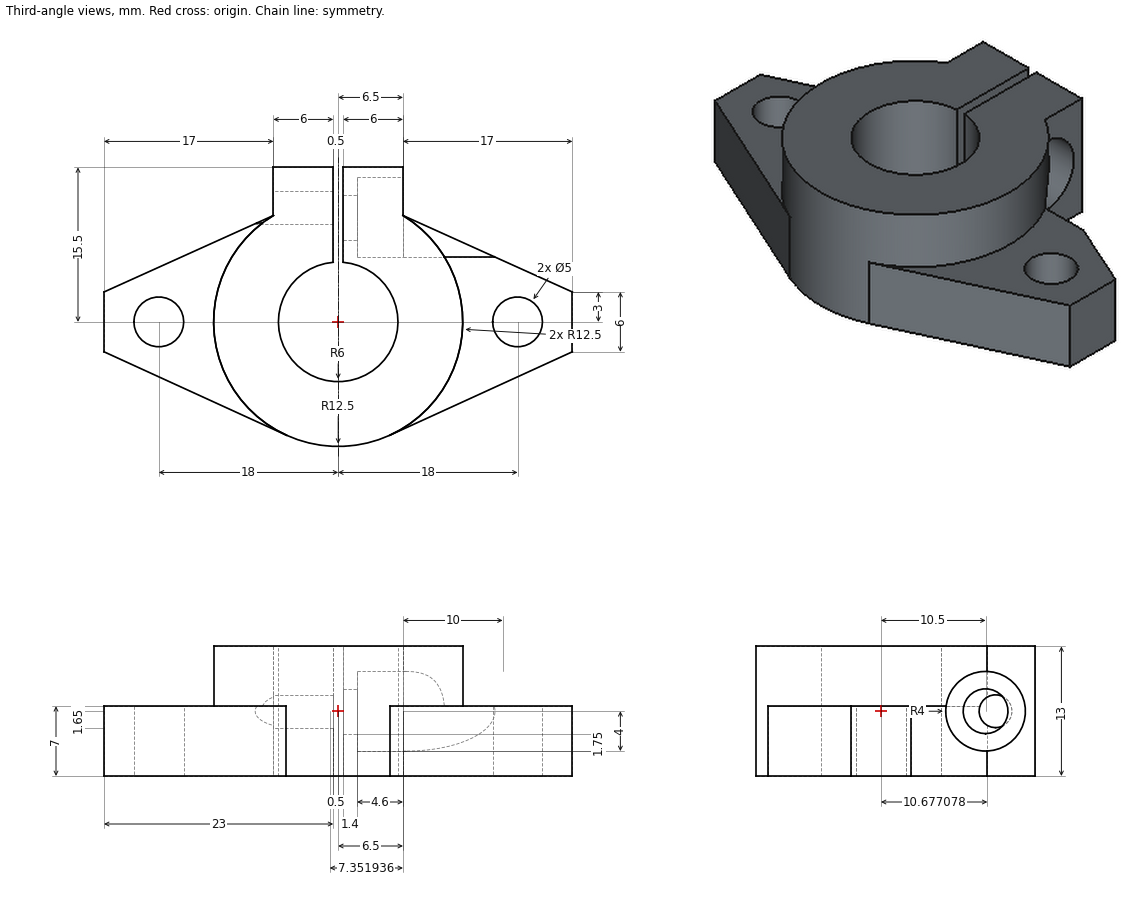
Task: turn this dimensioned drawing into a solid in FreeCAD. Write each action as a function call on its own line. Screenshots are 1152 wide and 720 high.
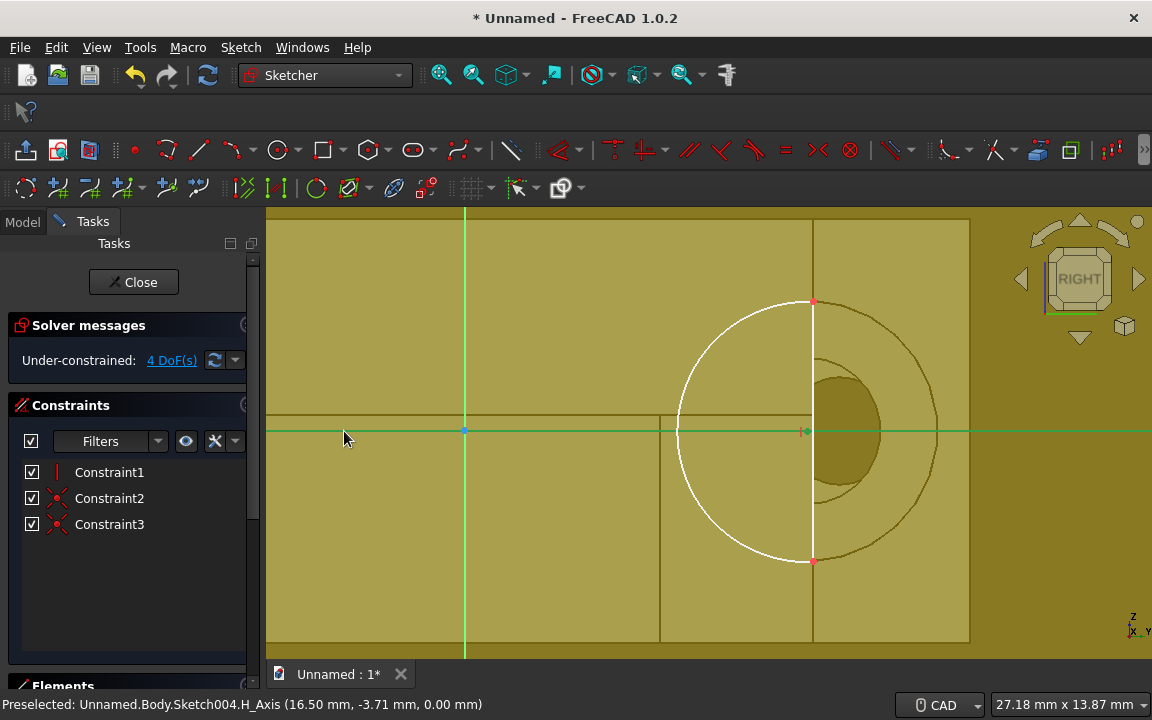
click(614, 150)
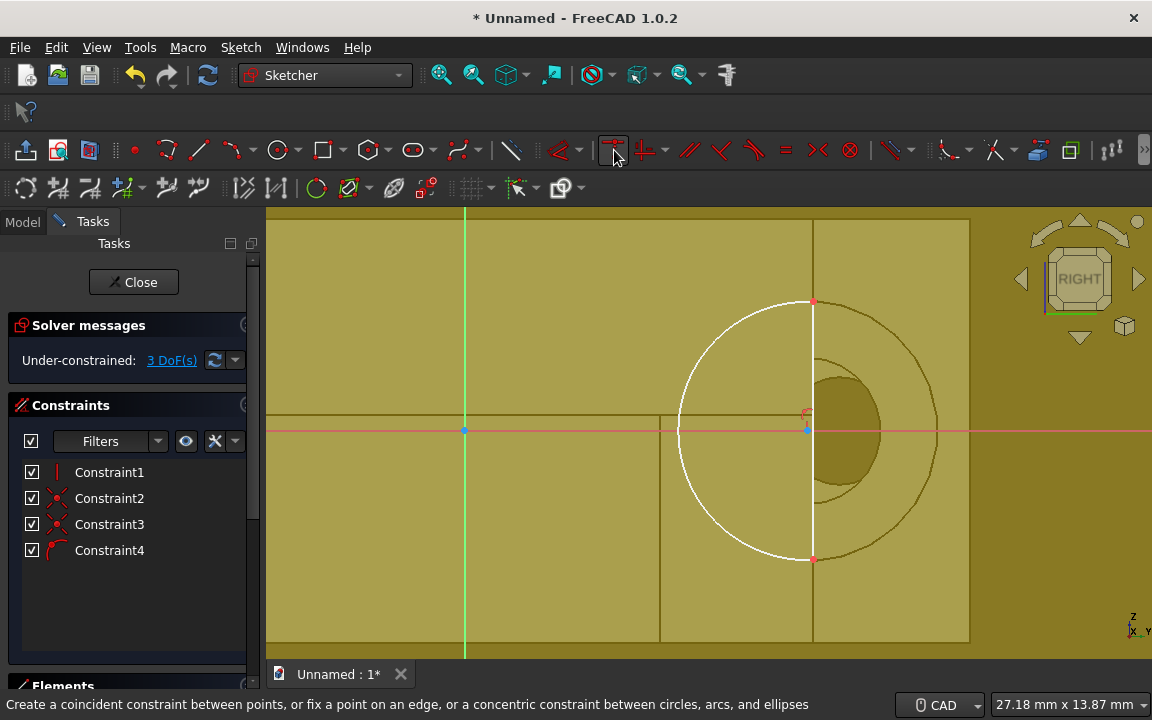
click(558, 150)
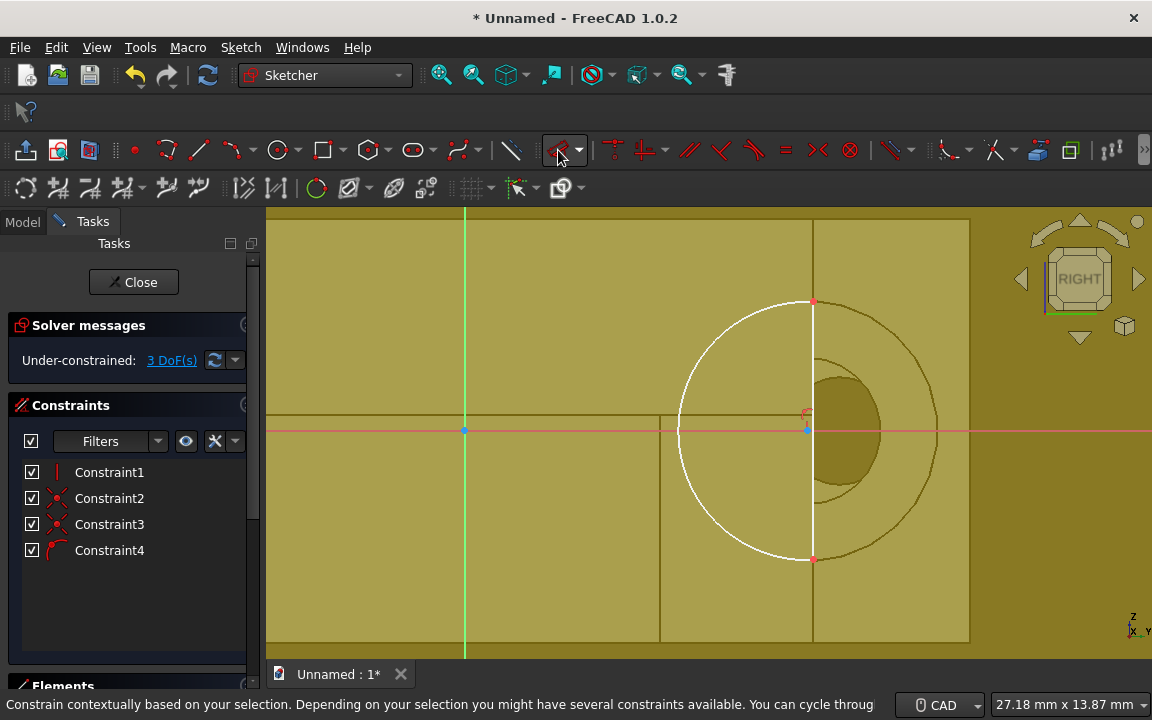
click(704, 353)
click(678, 334)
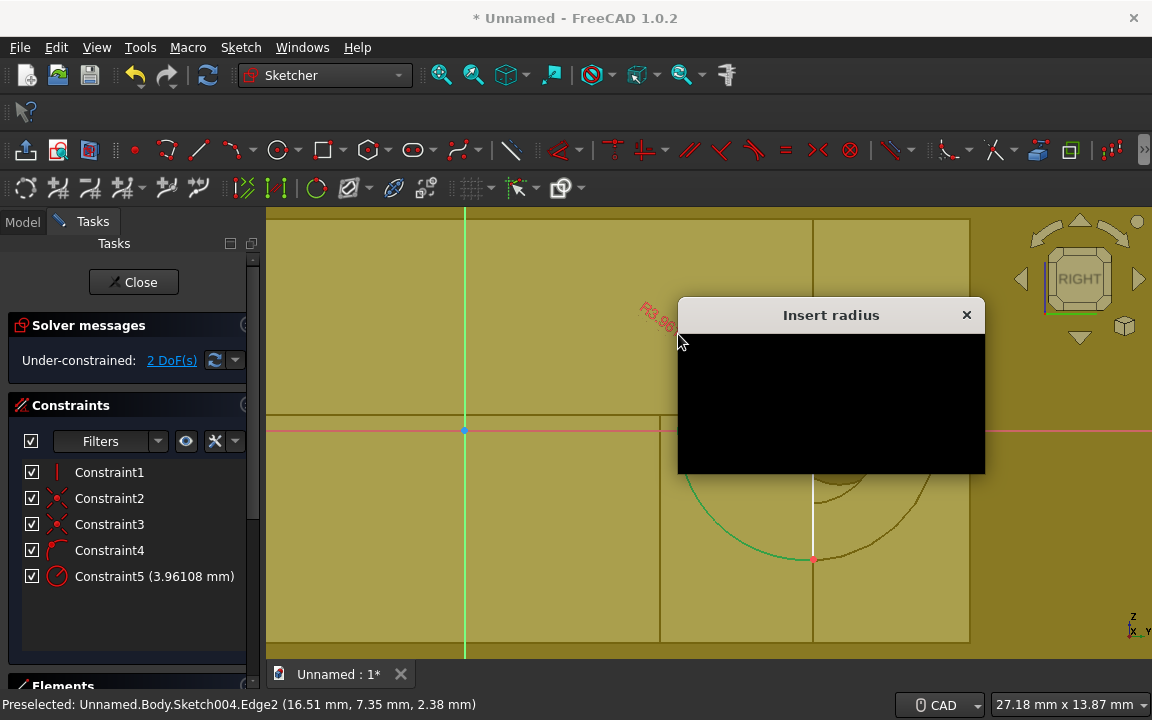
text(4)
key(Return)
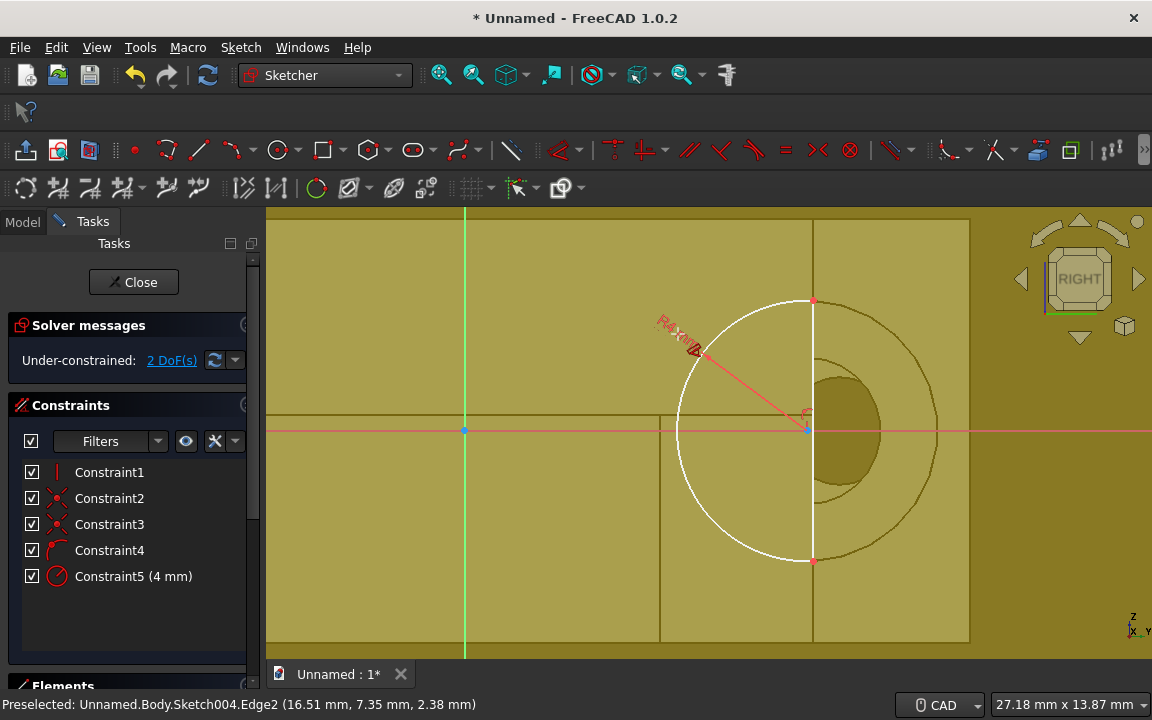
click(807, 431)
click(636, 465)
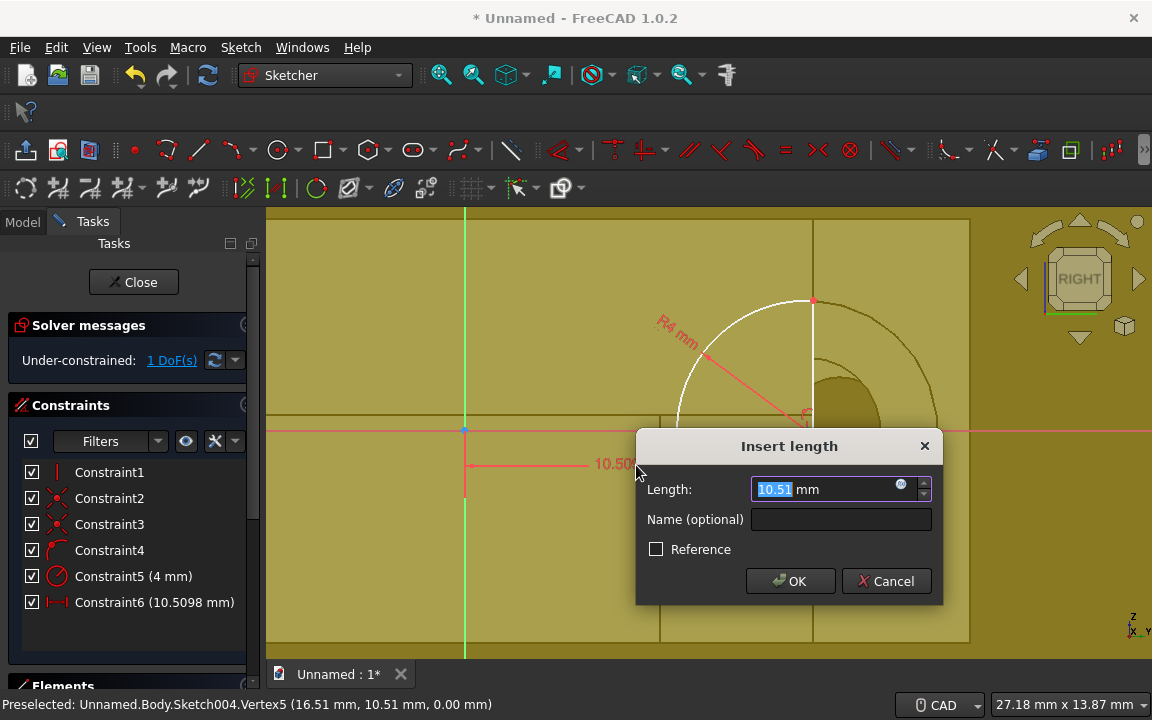
text(10.5)
key(Return)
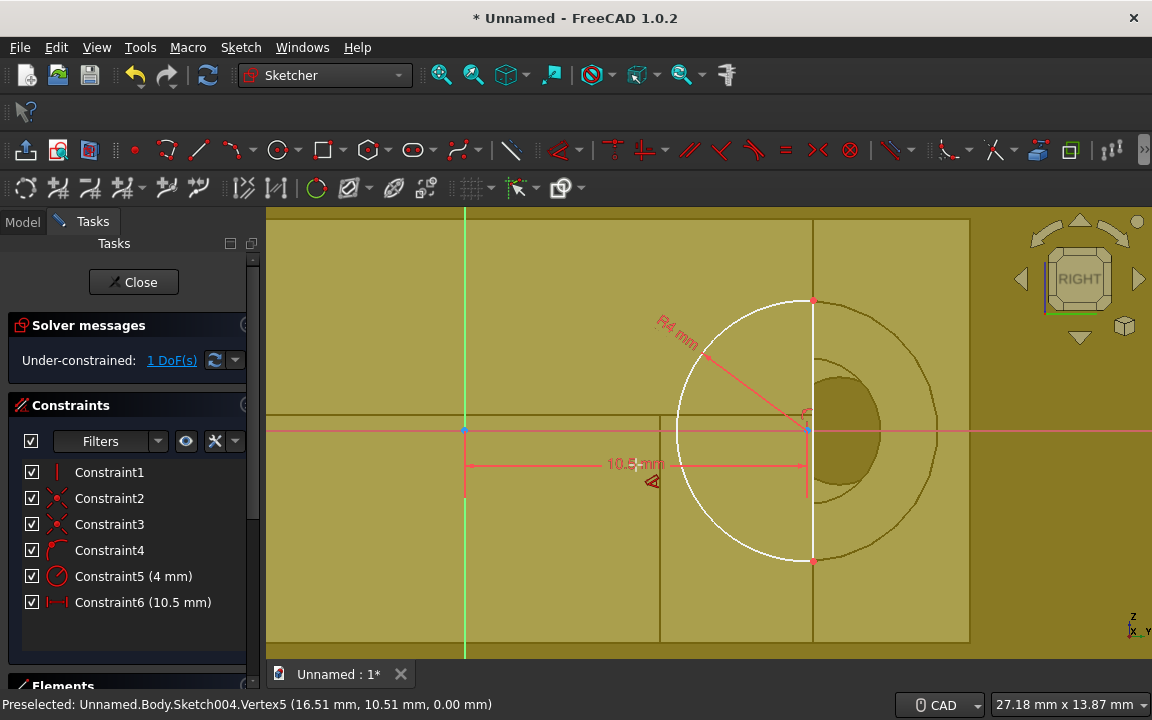
click(813, 561)
click(639, 595)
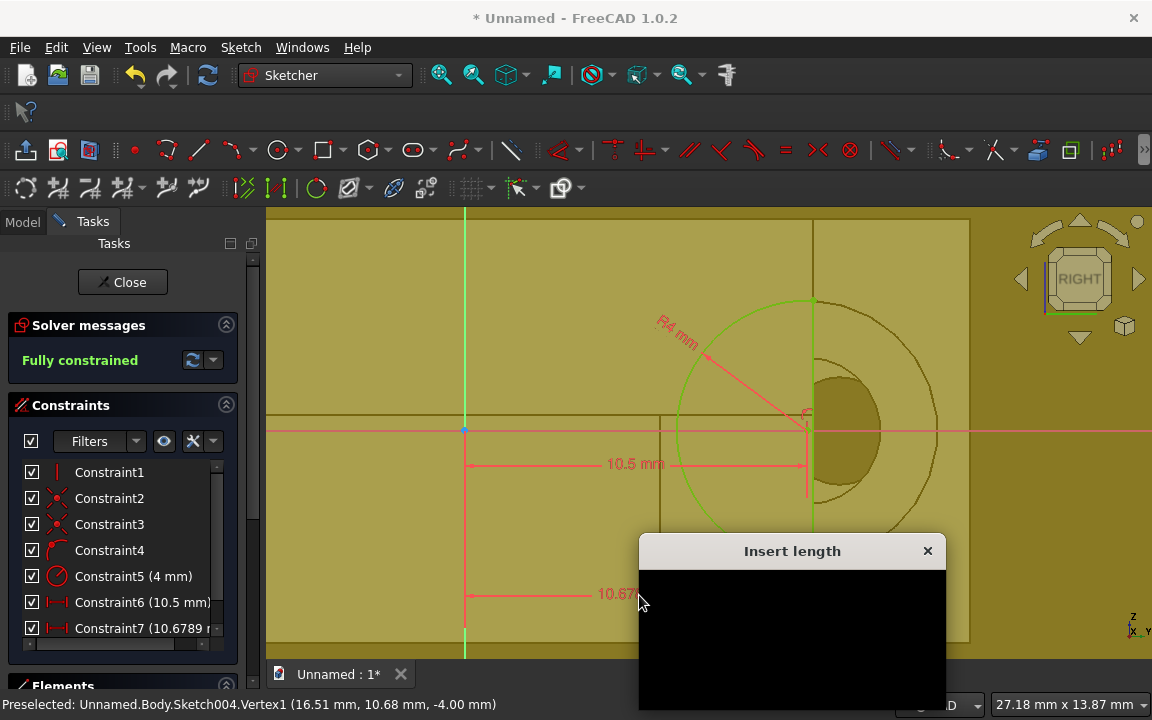
text(10.677078)
key(Return)
key(Escape)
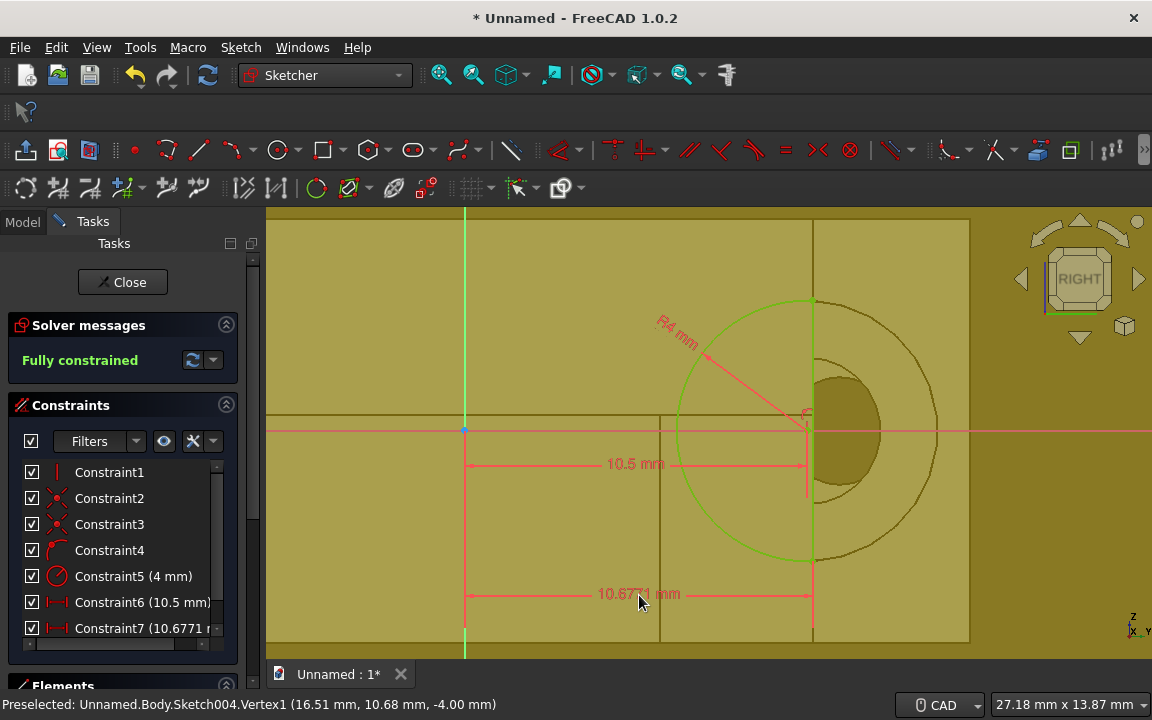
click(123, 282)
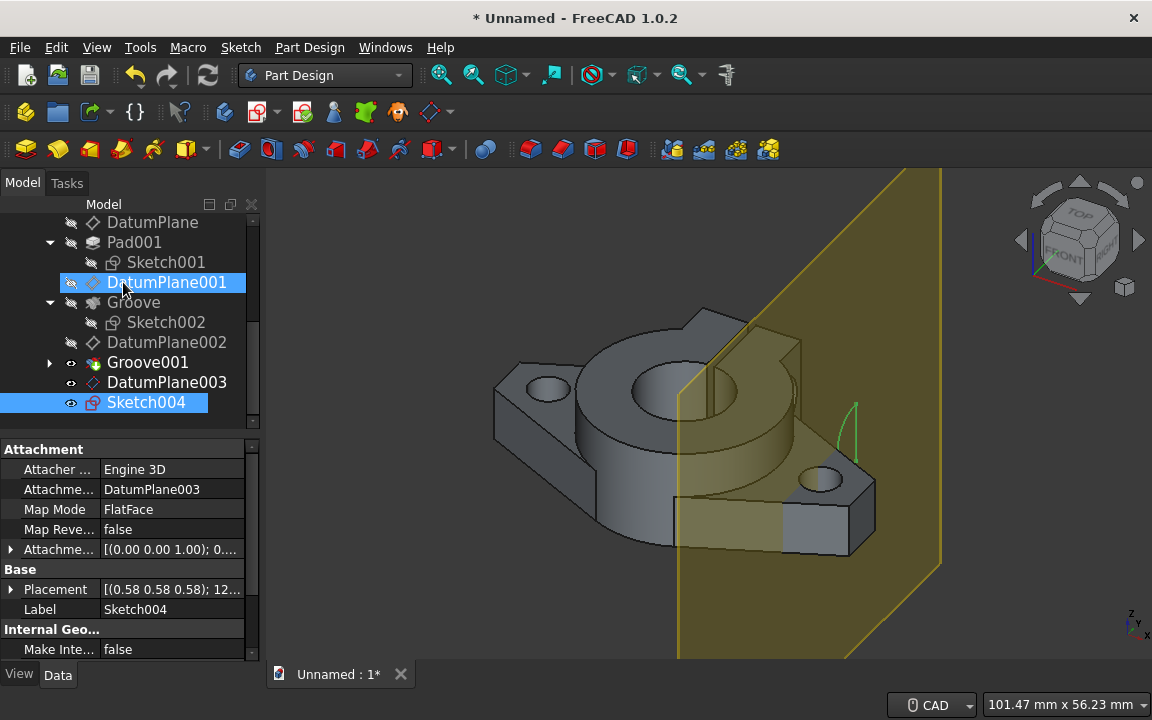
click(240, 150)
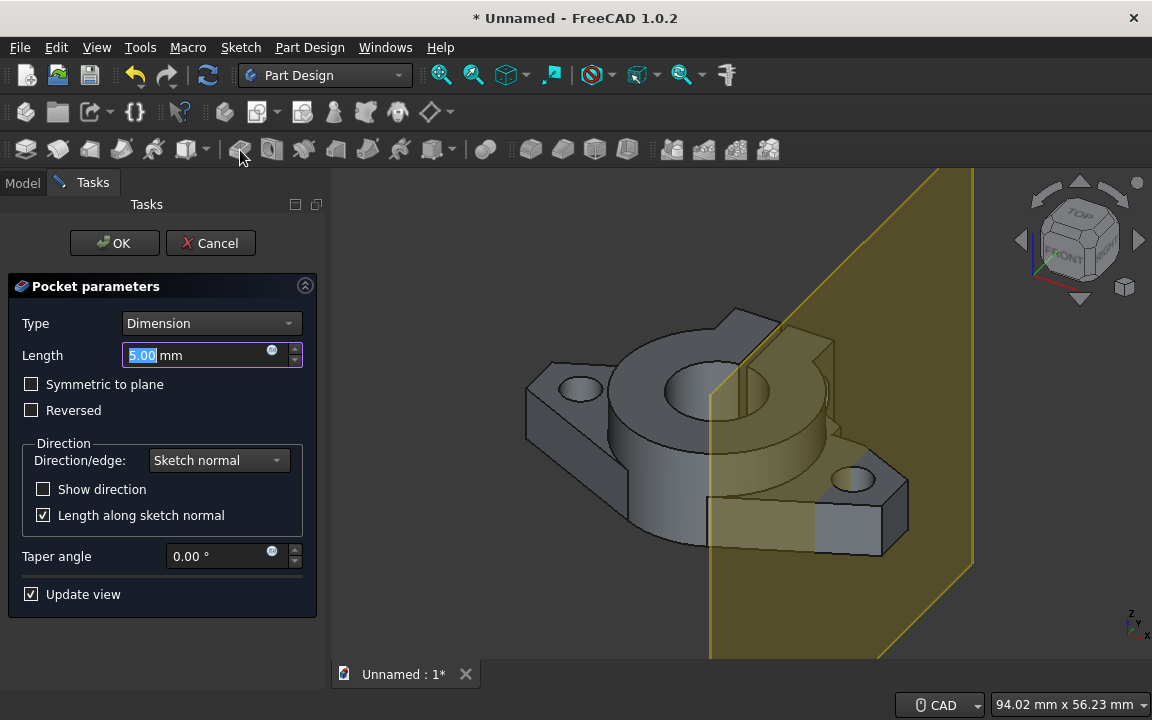
text(10)
key(Tab)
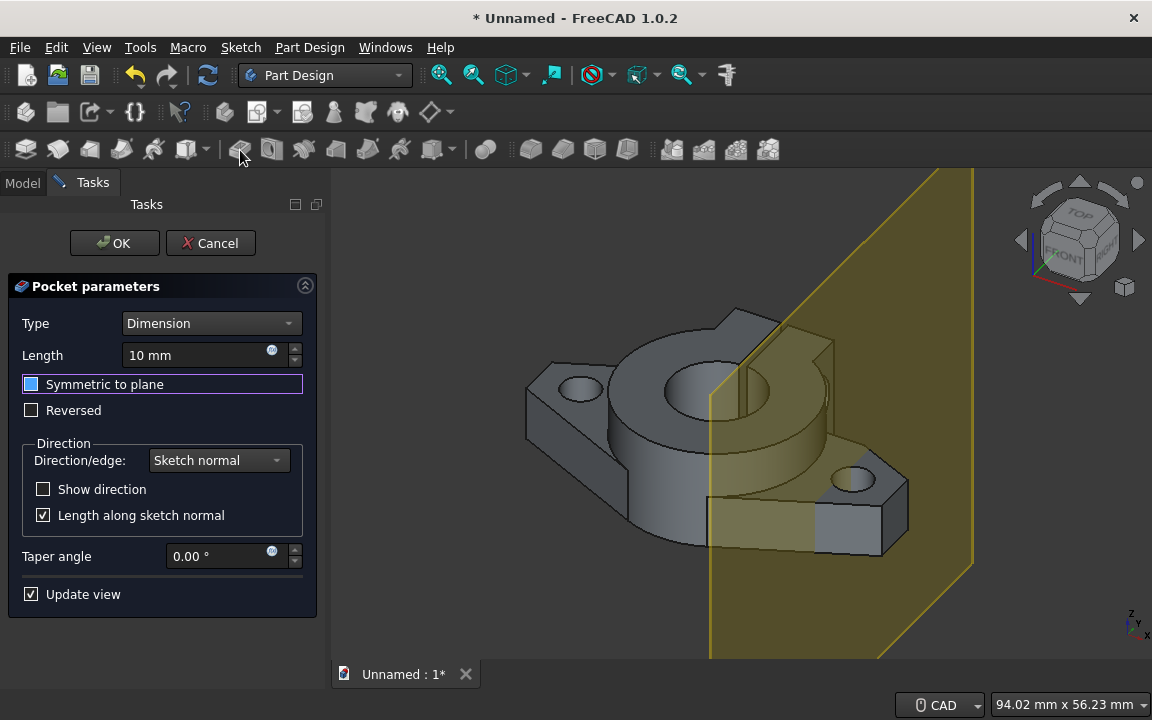
click(115, 243)